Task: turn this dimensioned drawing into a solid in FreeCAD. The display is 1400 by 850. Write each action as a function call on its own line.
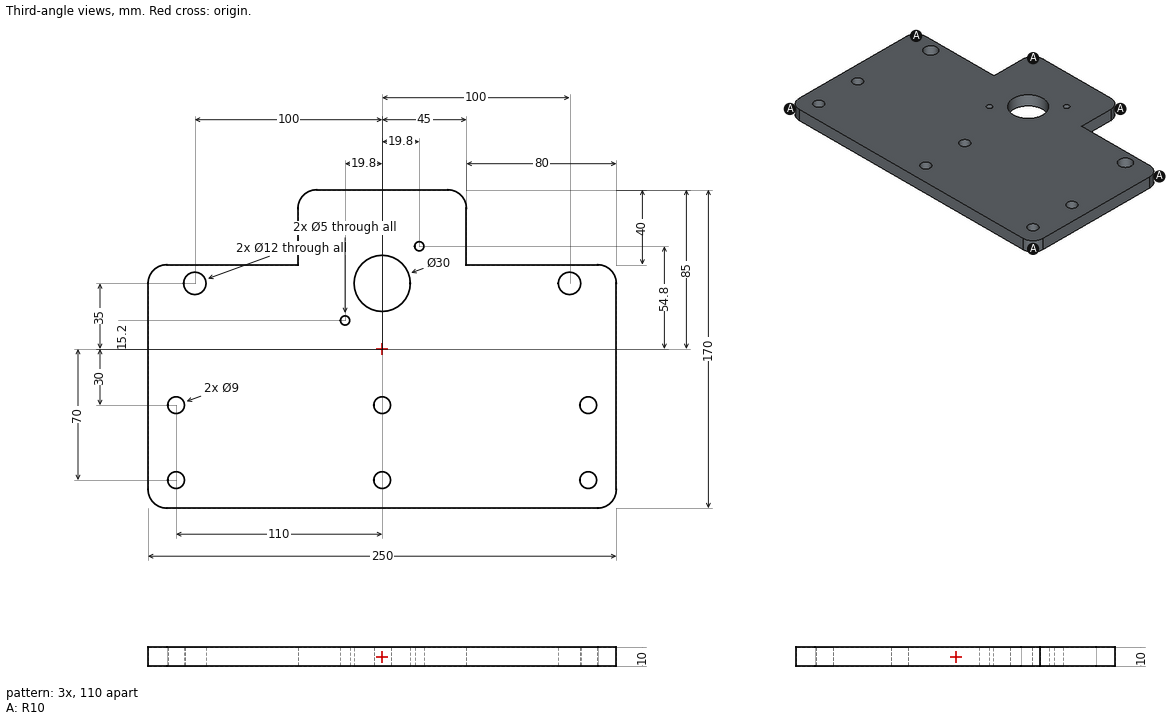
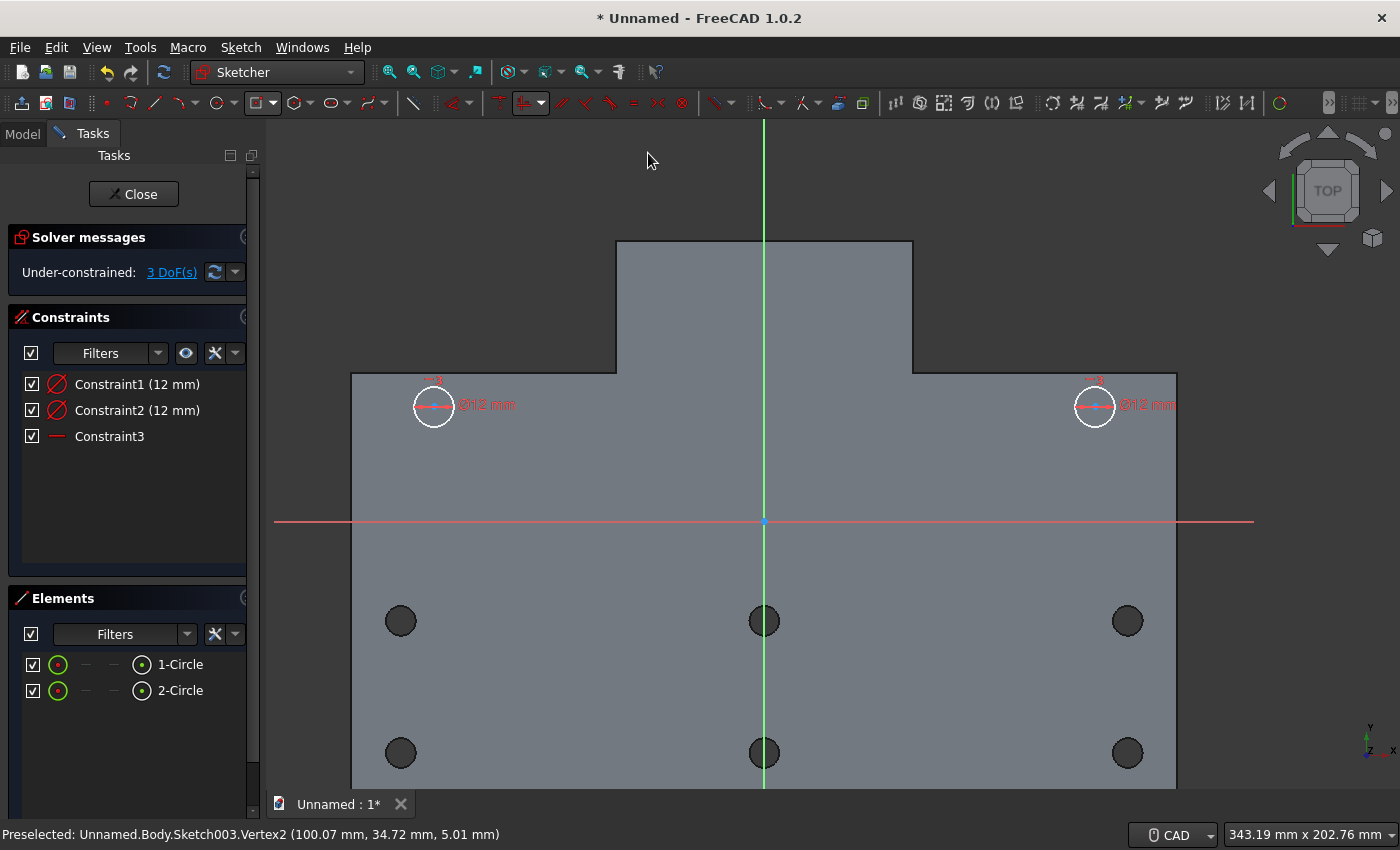
click(452, 104)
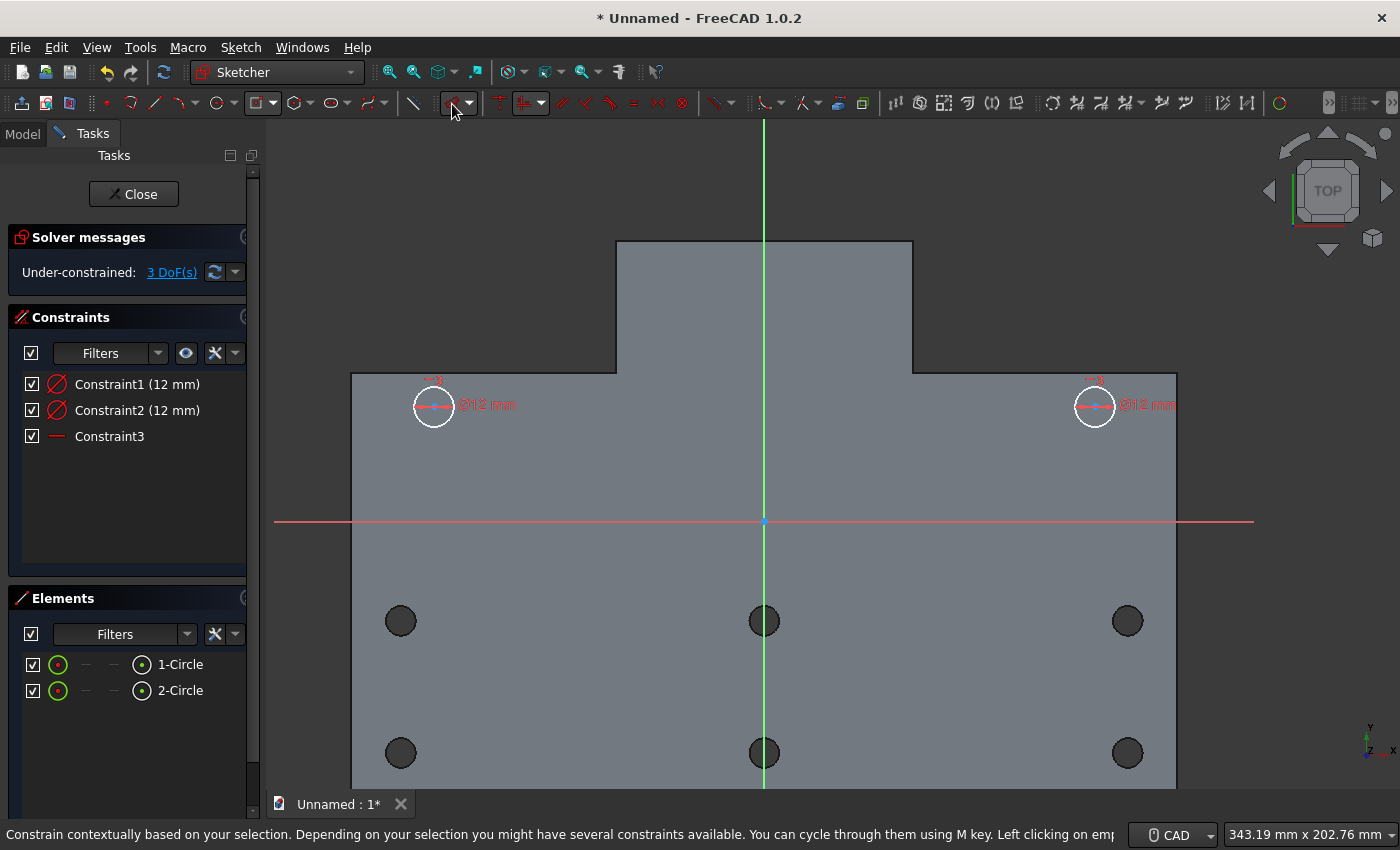
click(434, 407)
click(400, 464)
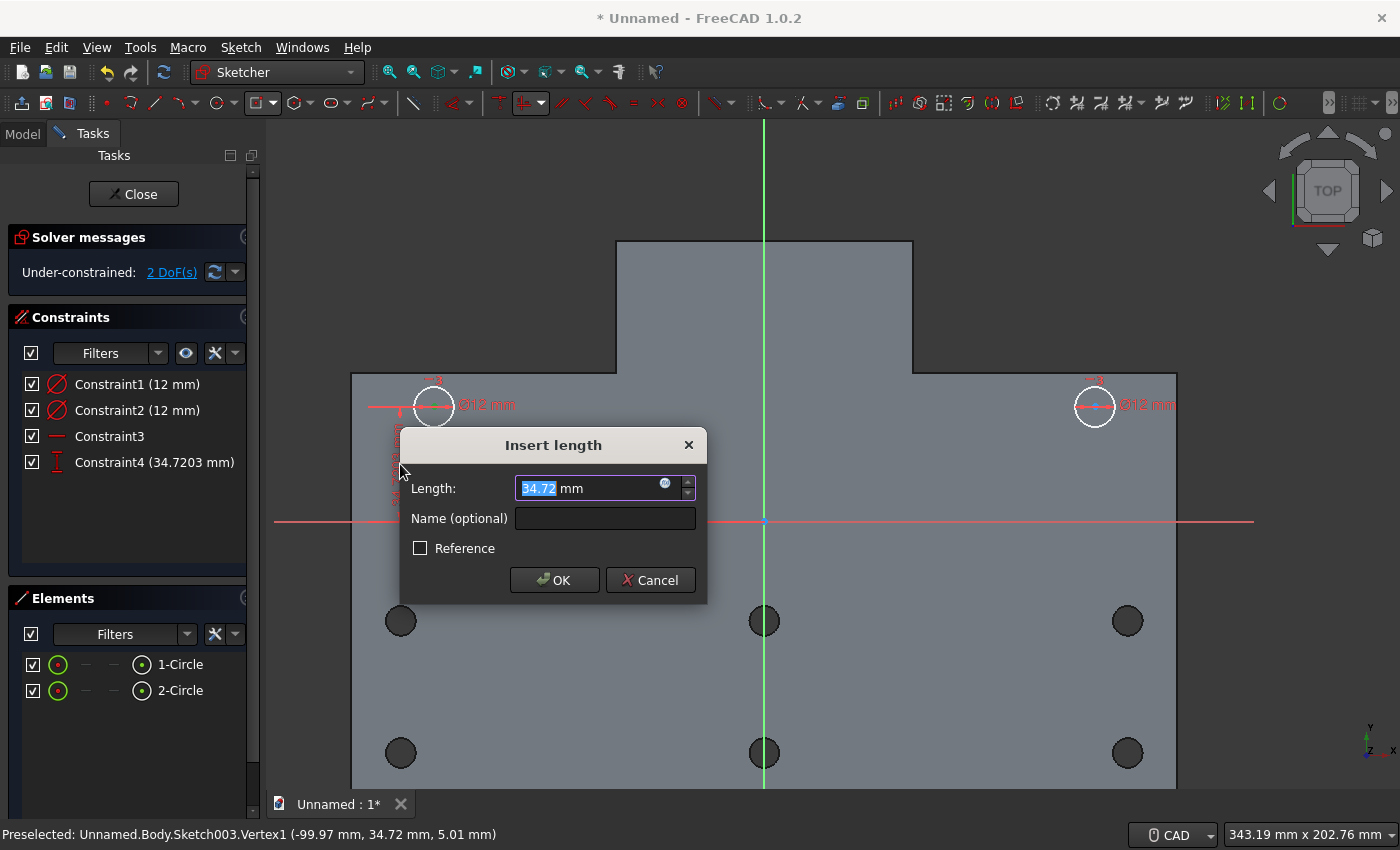
text(35)
key(Return)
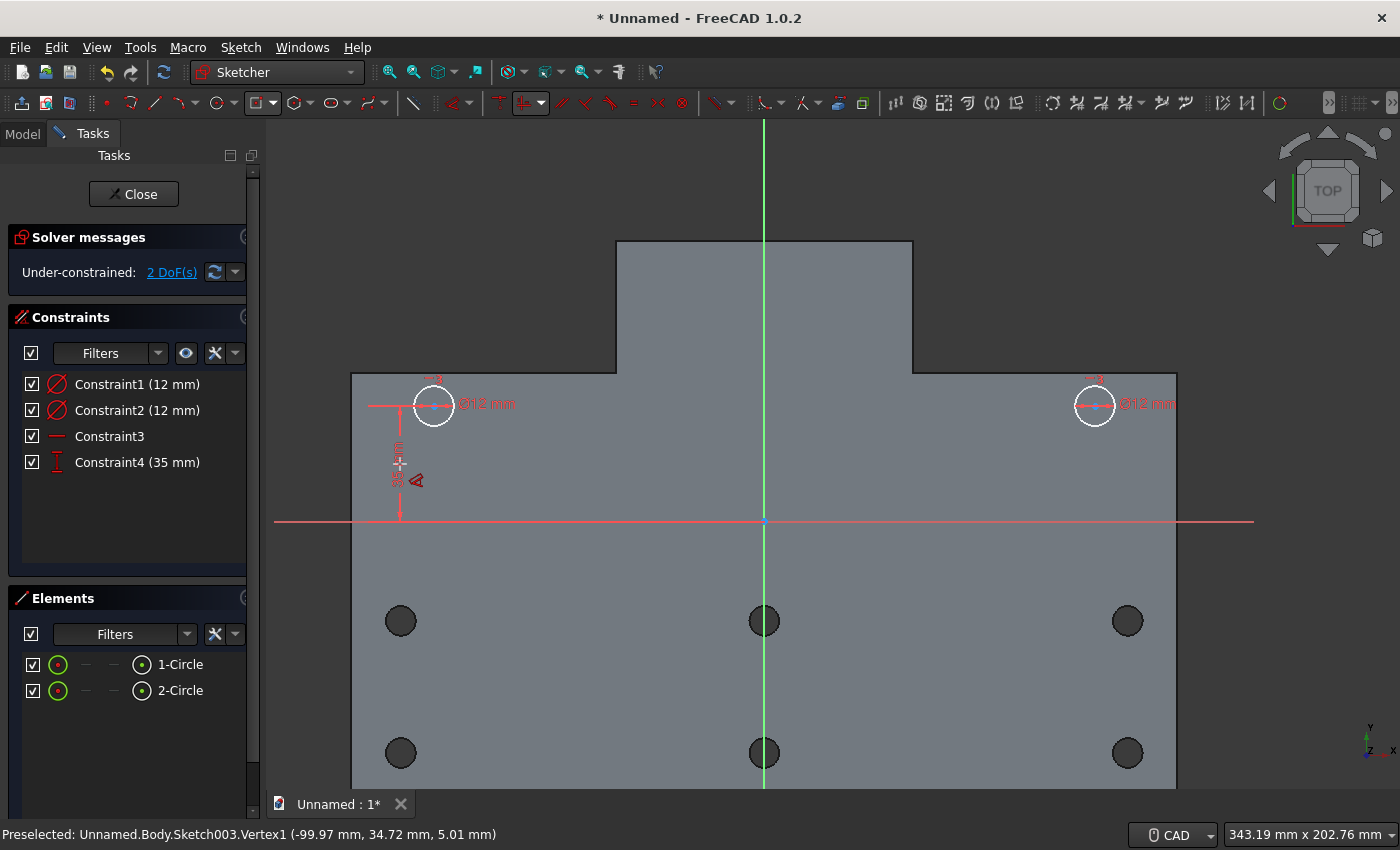
click(434, 406)
click(599, 556)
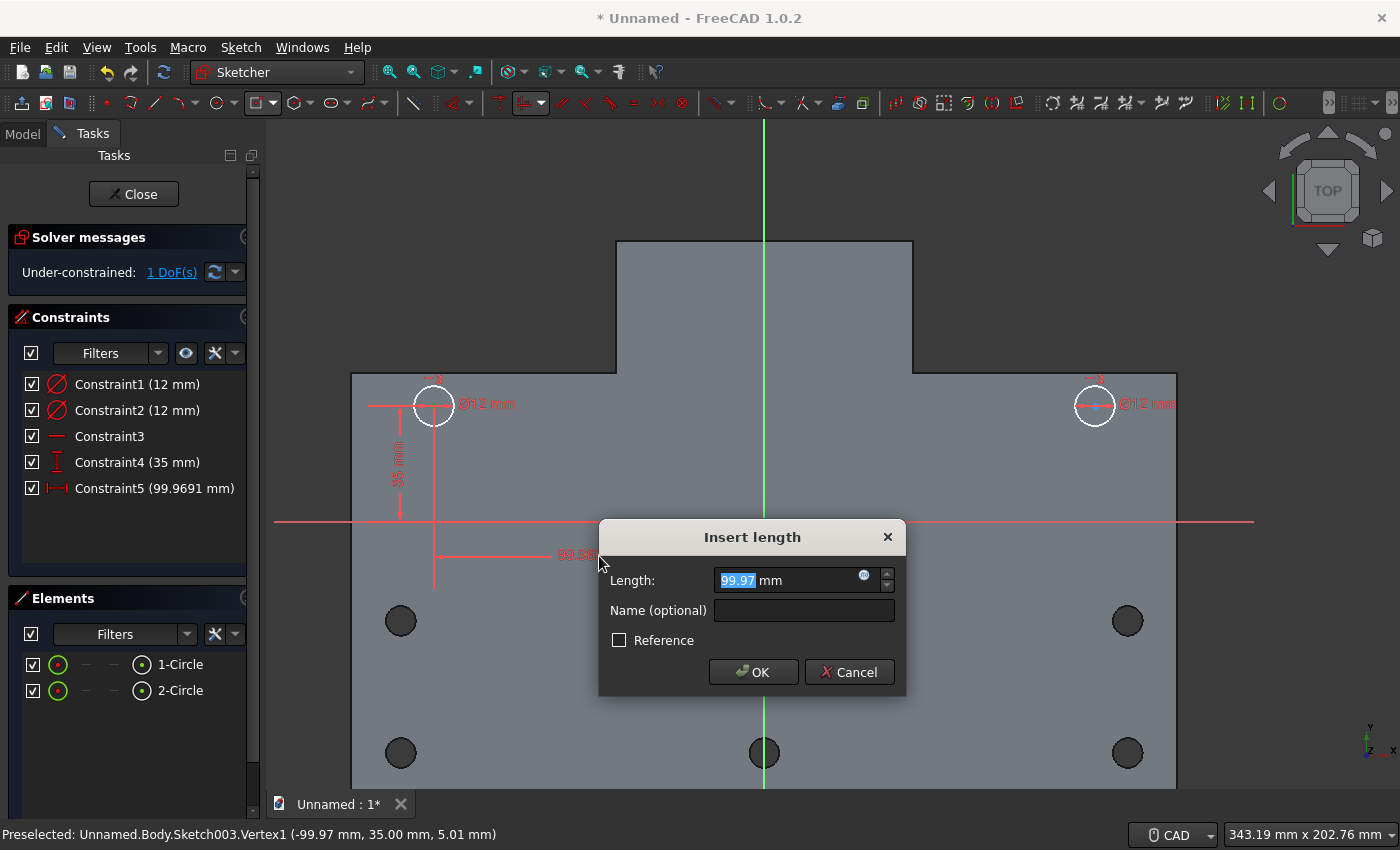
text(100)
key(Return)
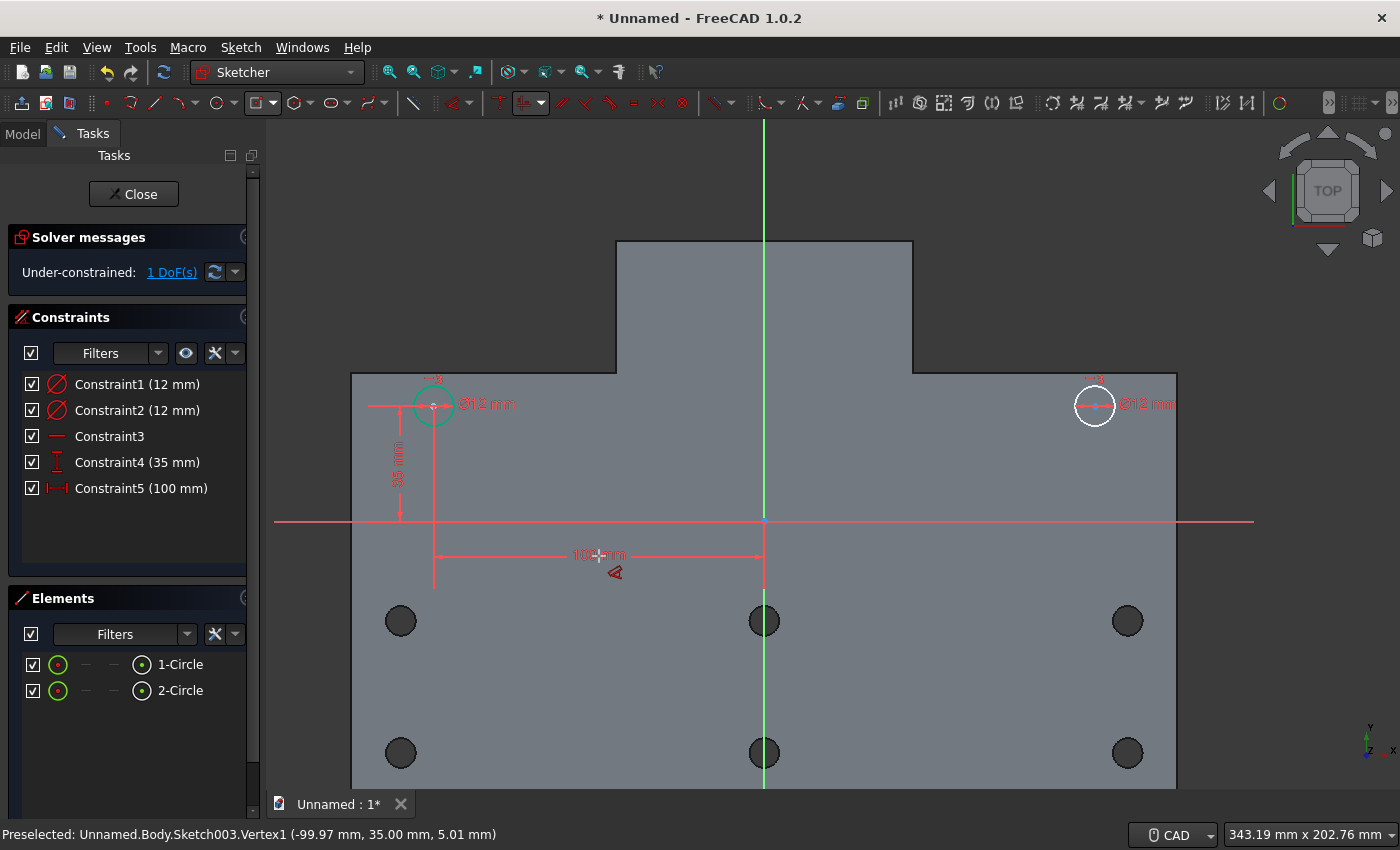
click(1095, 406)
click(930, 556)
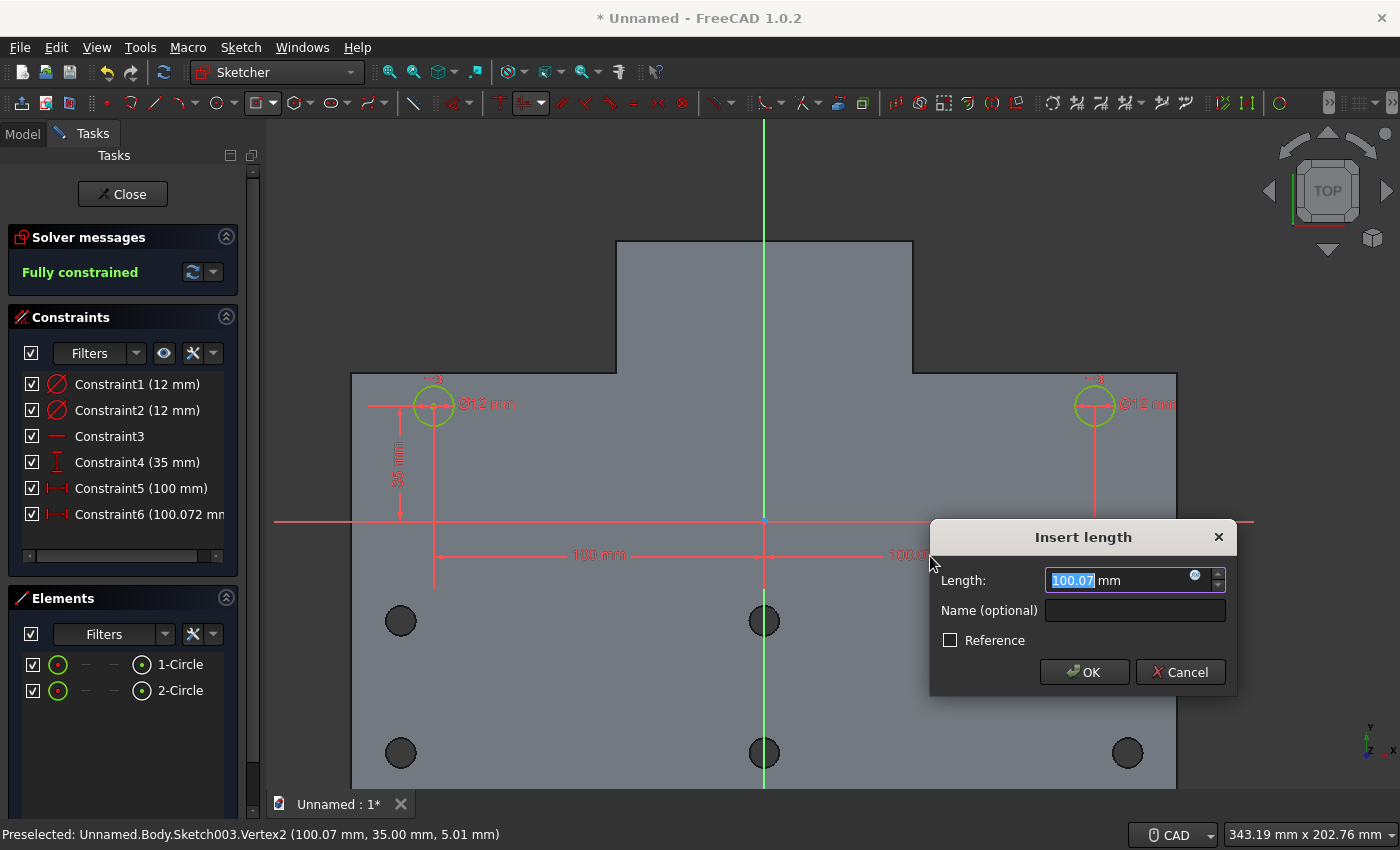
text(100)
key(Return)
key(Escape)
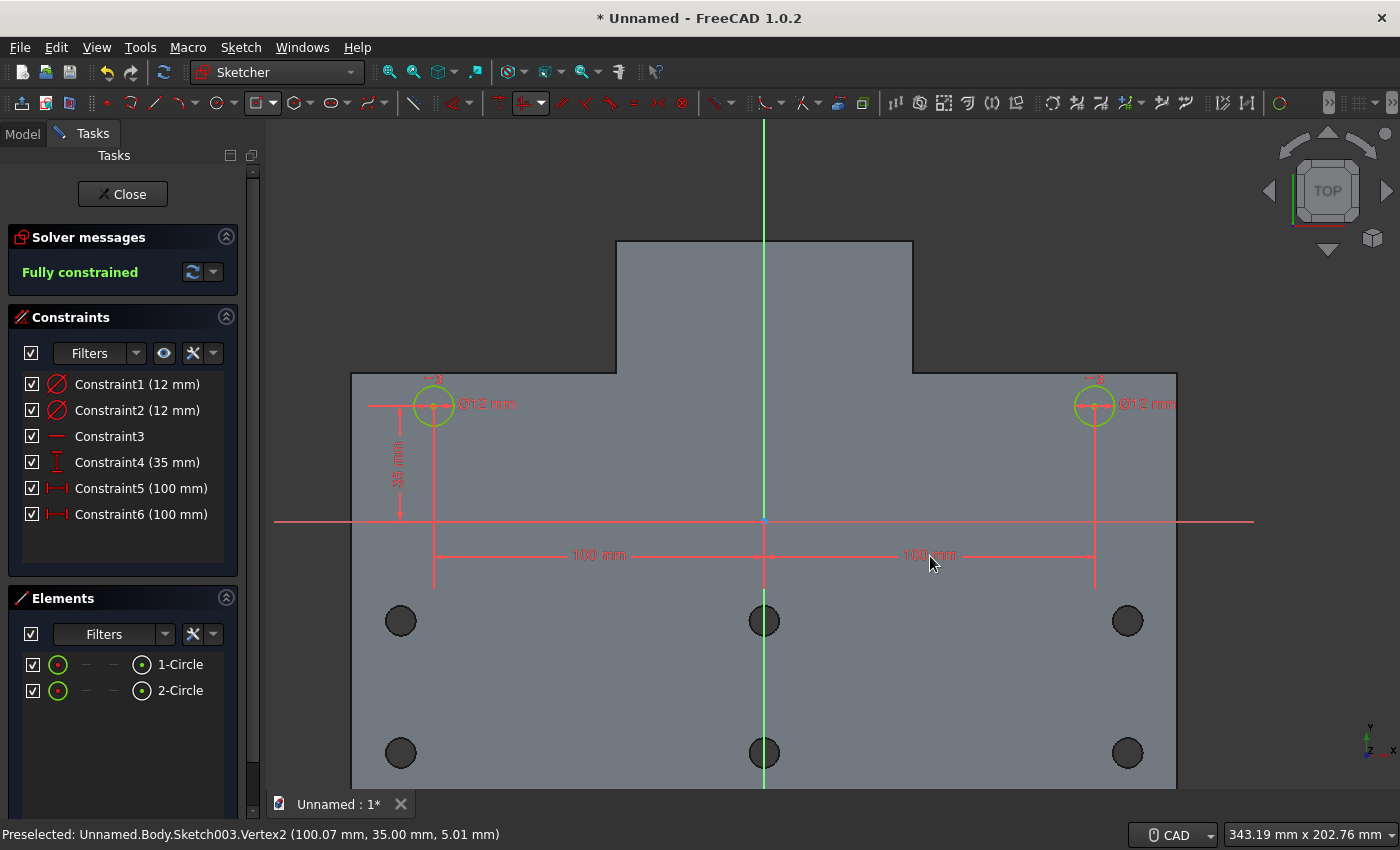
click(123, 194)